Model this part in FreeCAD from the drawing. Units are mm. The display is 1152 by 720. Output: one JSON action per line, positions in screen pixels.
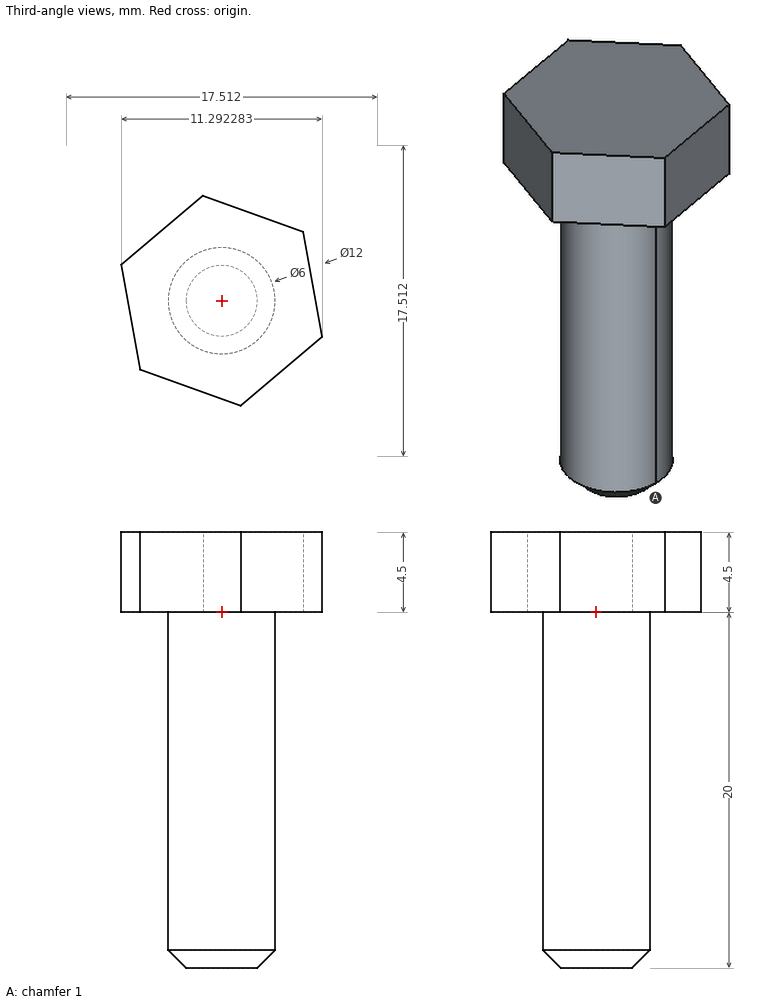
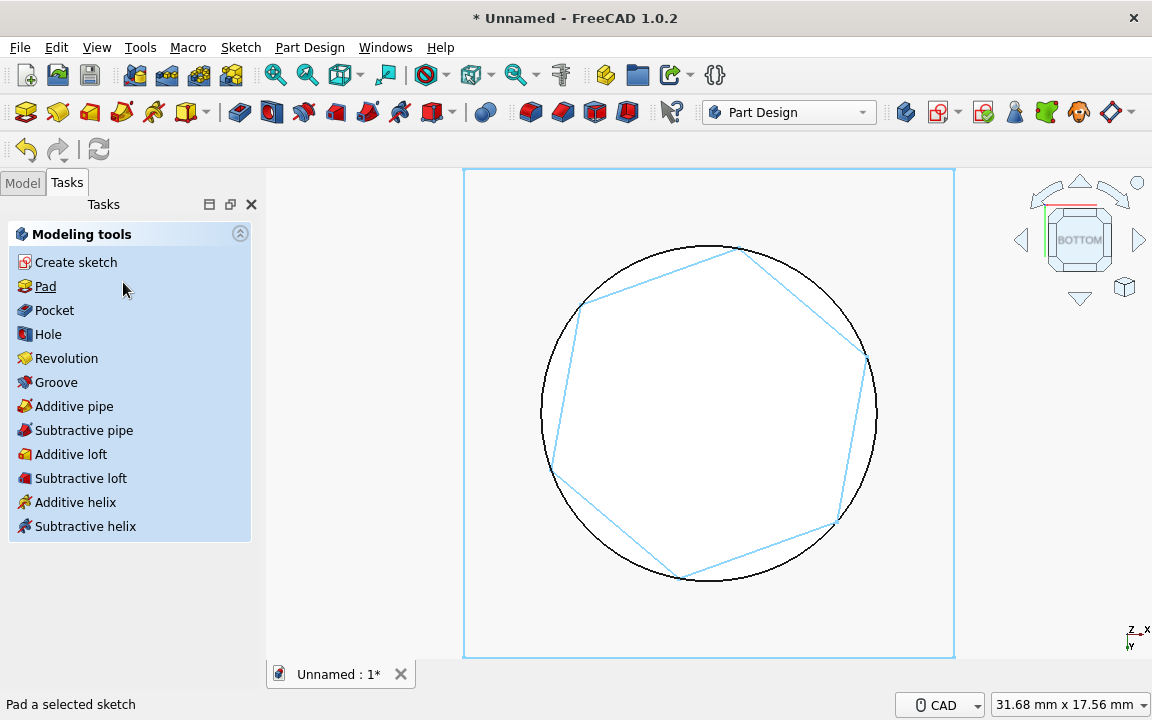
{"action": "left_click", "coordinate": [240, 112]}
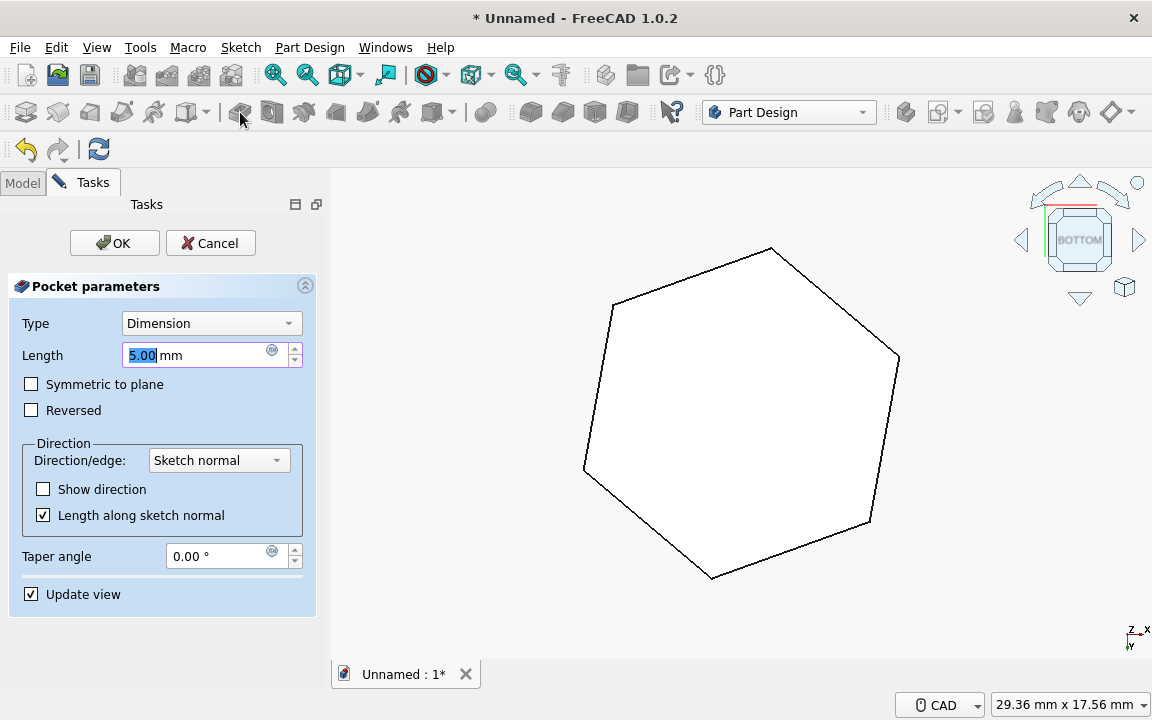
{"action": "type", "text": "4.5"}
{"action": "key", "text": "Tab"}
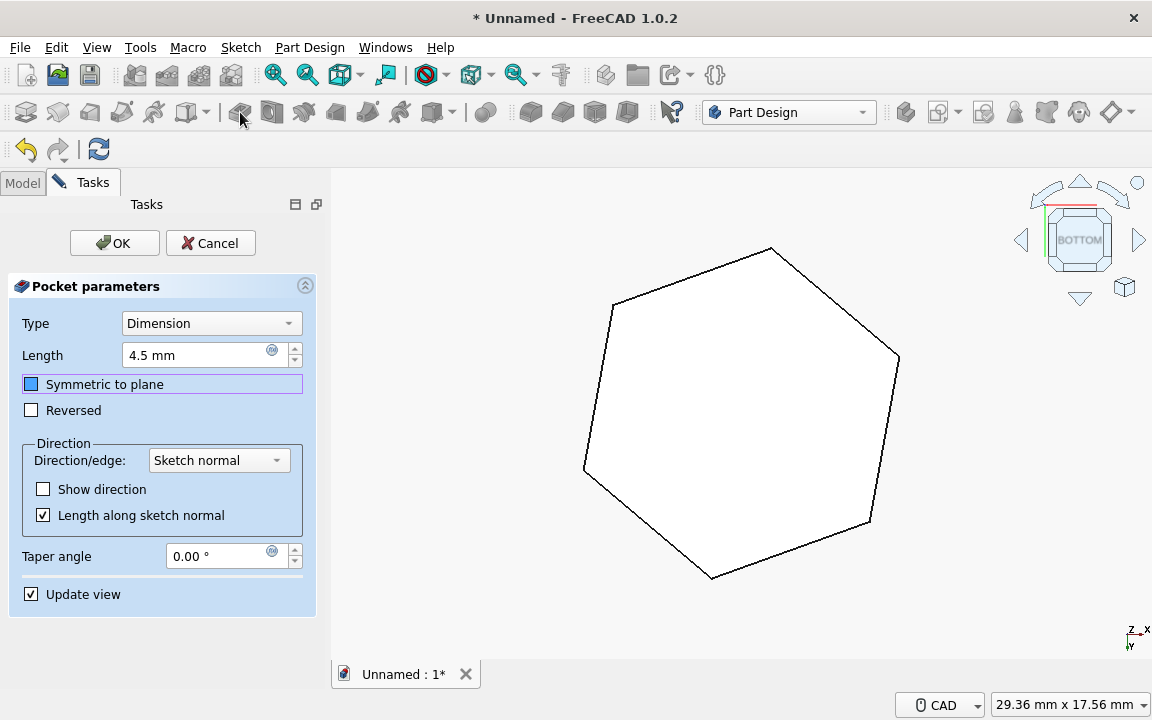
{"action": "left_click", "coordinate": [115, 243]}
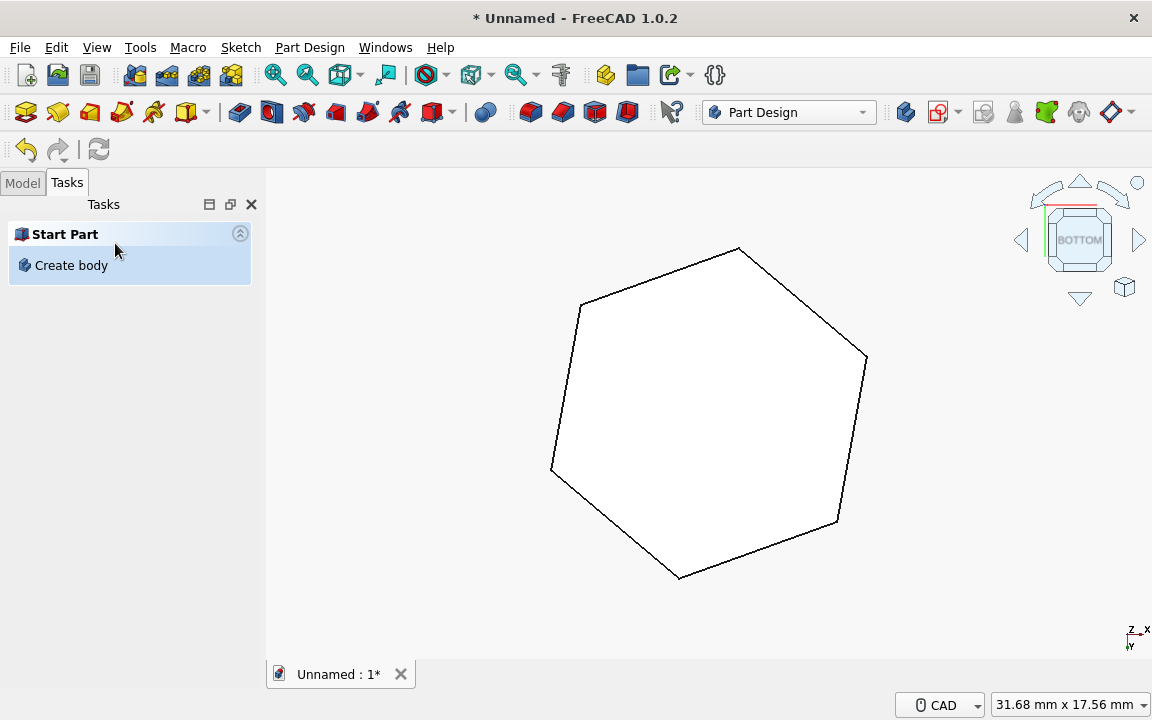
{"action": "left_click", "coordinate": [938, 112]}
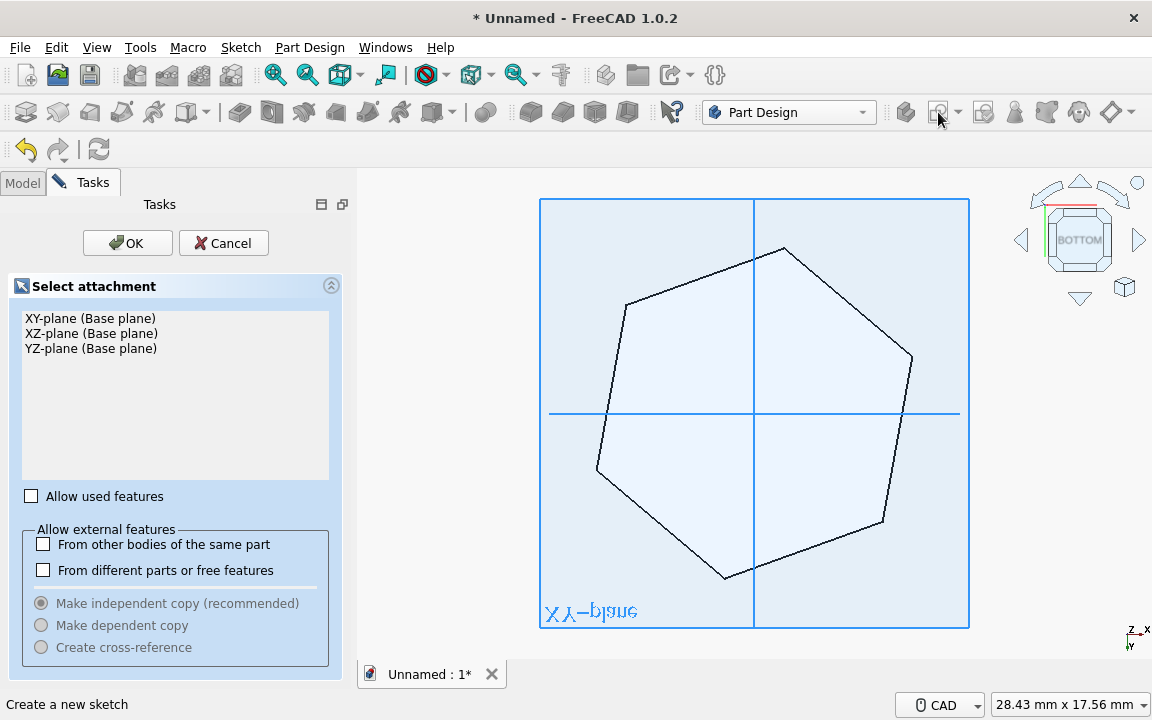
{"action": "left_click", "coordinate": [82, 318]}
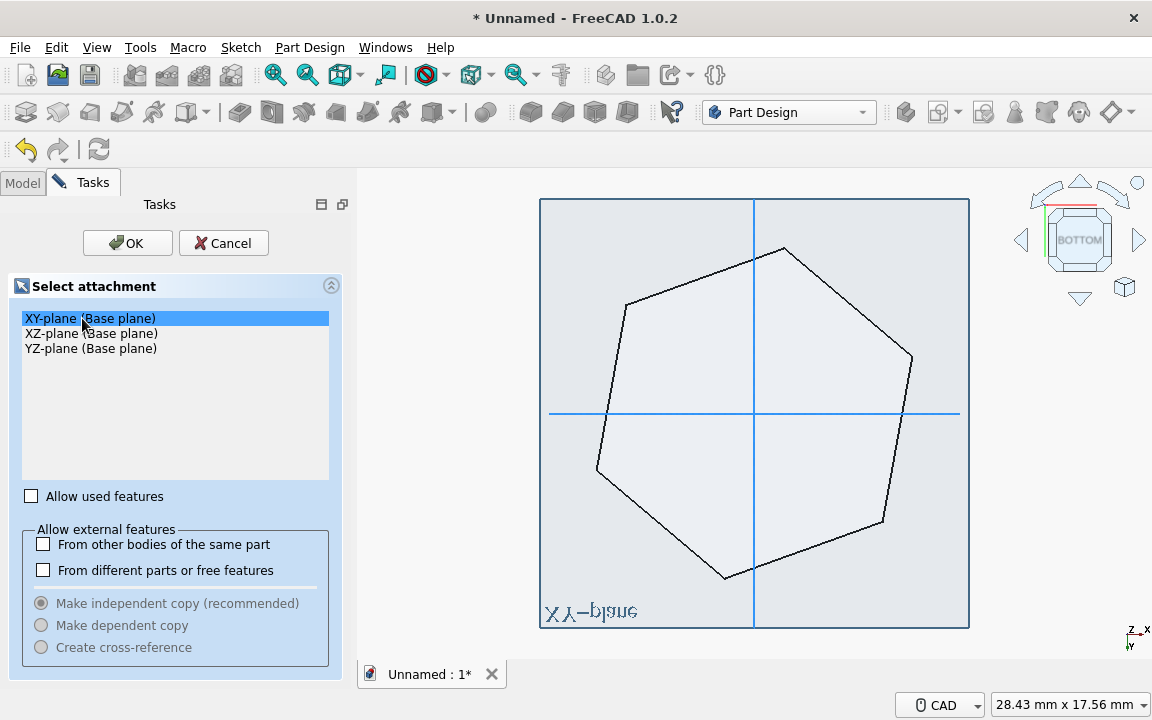
{"action": "left_click", "coordinate": [128, 243]}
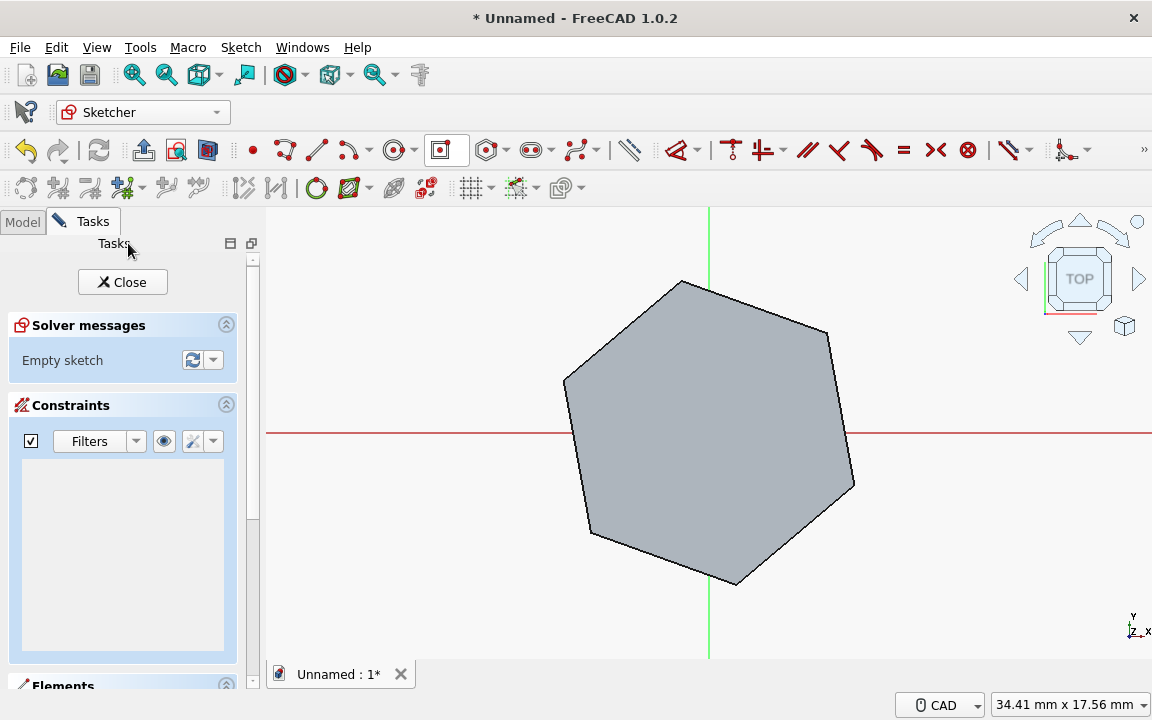
{"action": "key", "text": "q s"}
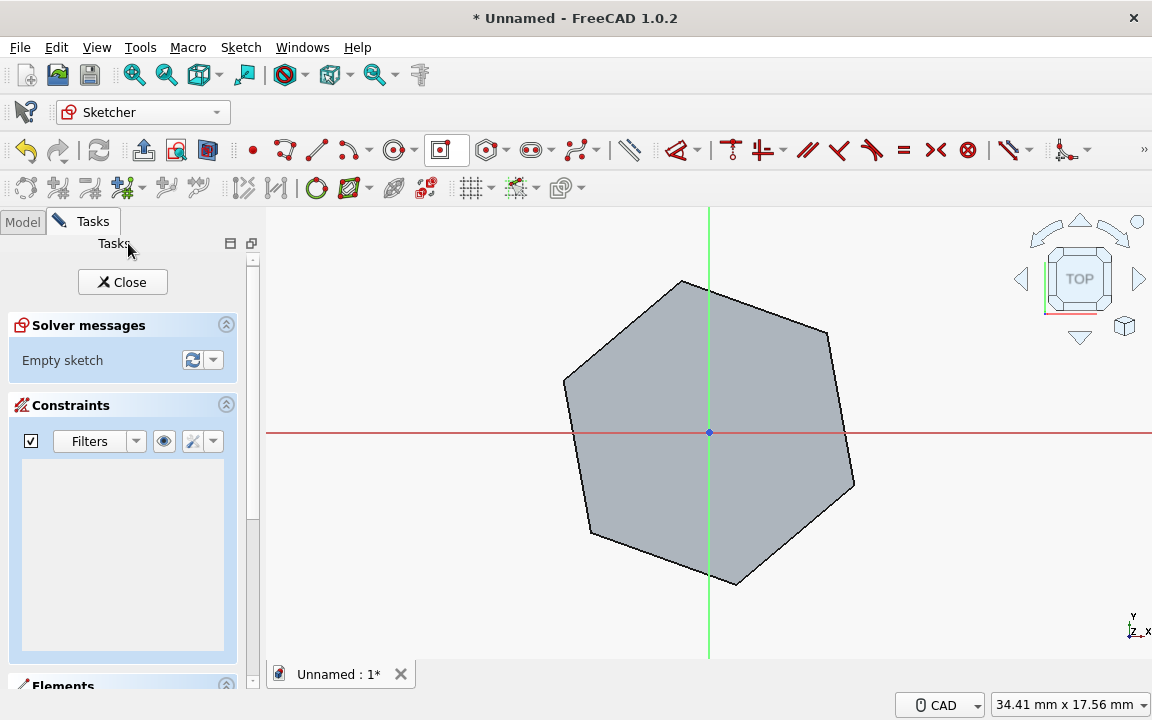
{"action": "scroll", "coordinate": [792, 433], "scroll_direction": "up", "scroll_amount": 3}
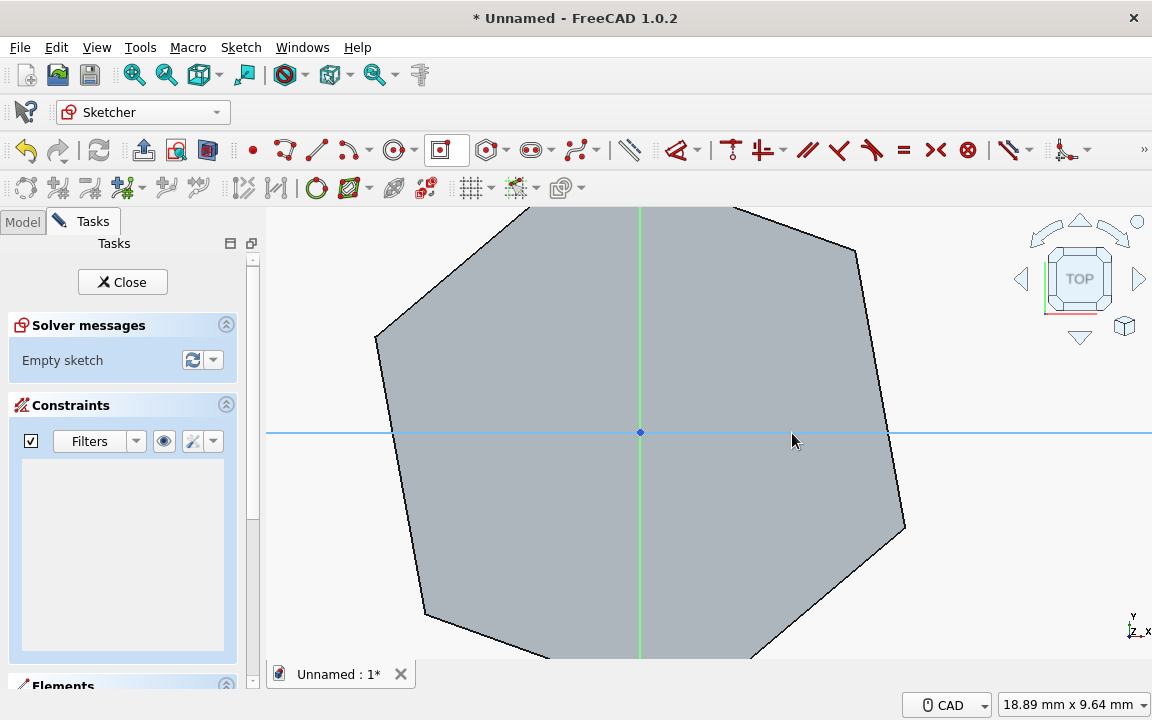
{"action": "key", "text": "g c"}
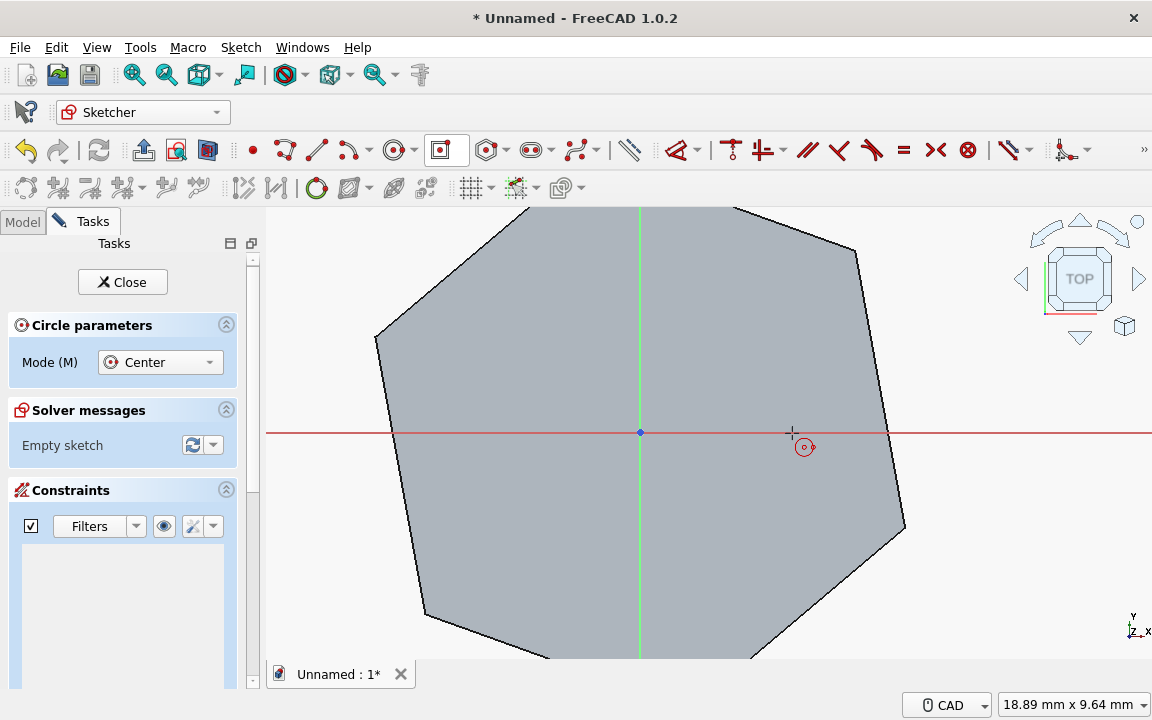
{"action": "left_click", "coordinate": [640, 433]}
{"action": "left_click", "coordinate": [740, 333]}
{"action": "key", "text": "Escape"}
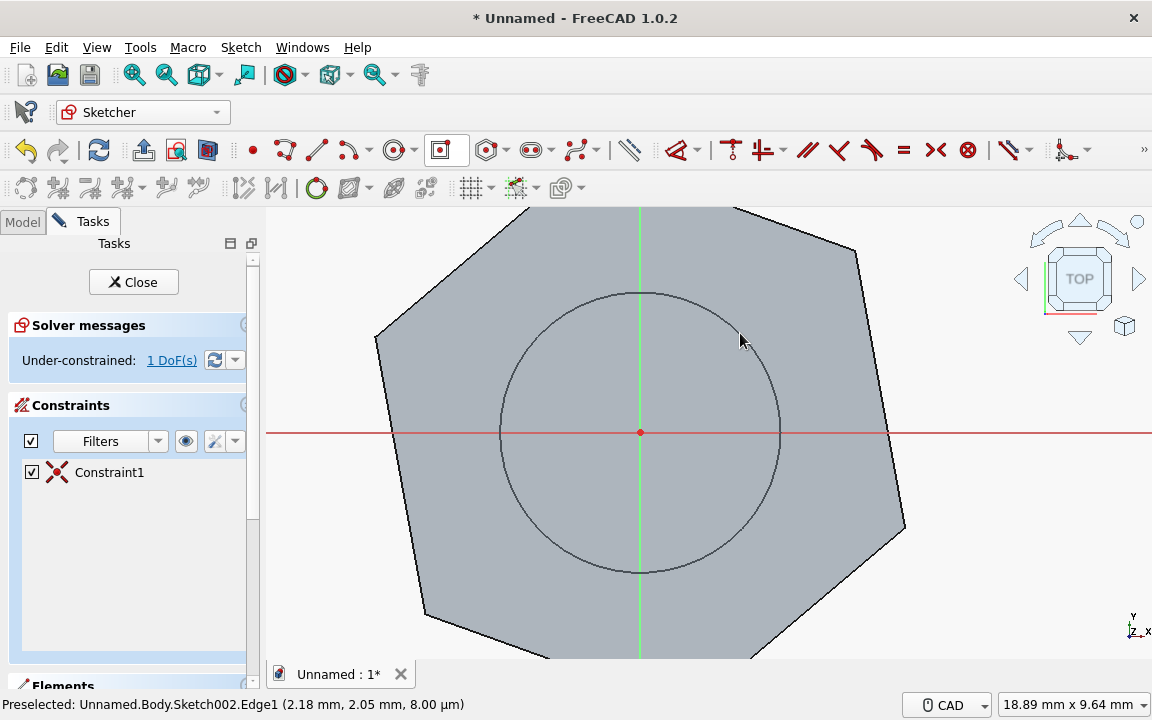
{"action": "key", "text": "d"}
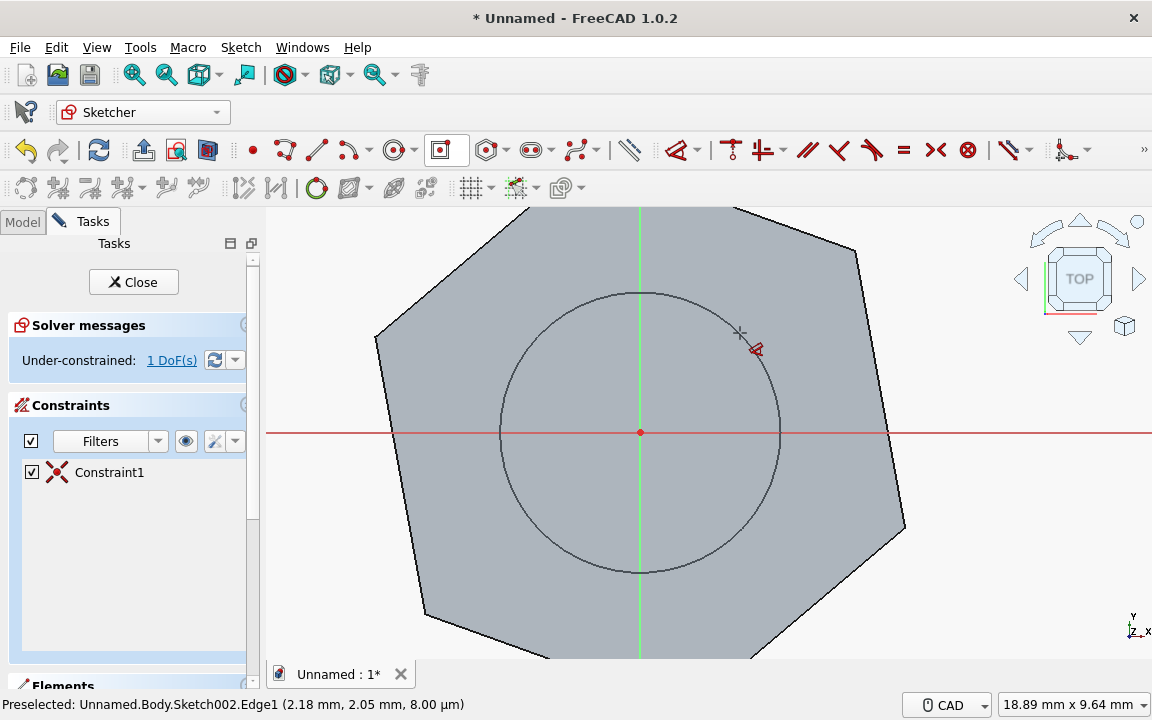
{"action": "left_click", "coordinate": [739, 333]}
{"action": "left_click", "coordinate": [762, 310]}